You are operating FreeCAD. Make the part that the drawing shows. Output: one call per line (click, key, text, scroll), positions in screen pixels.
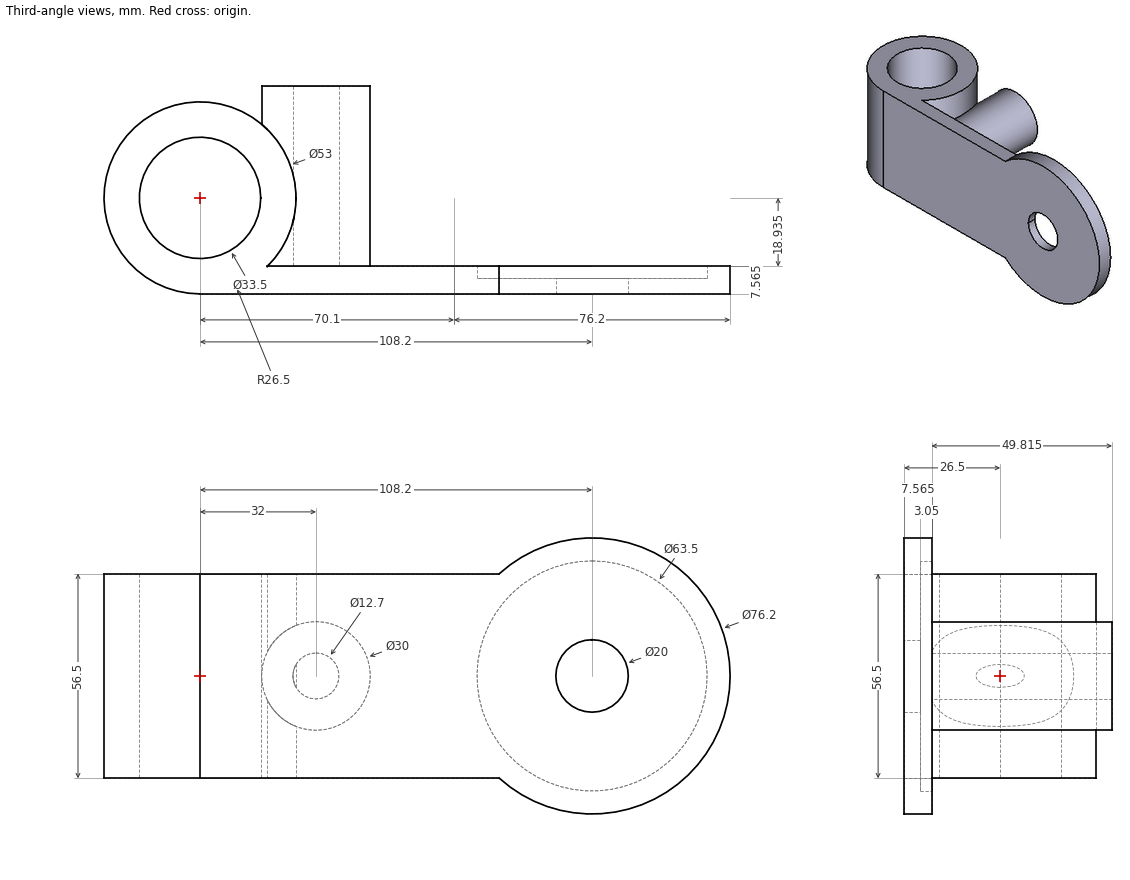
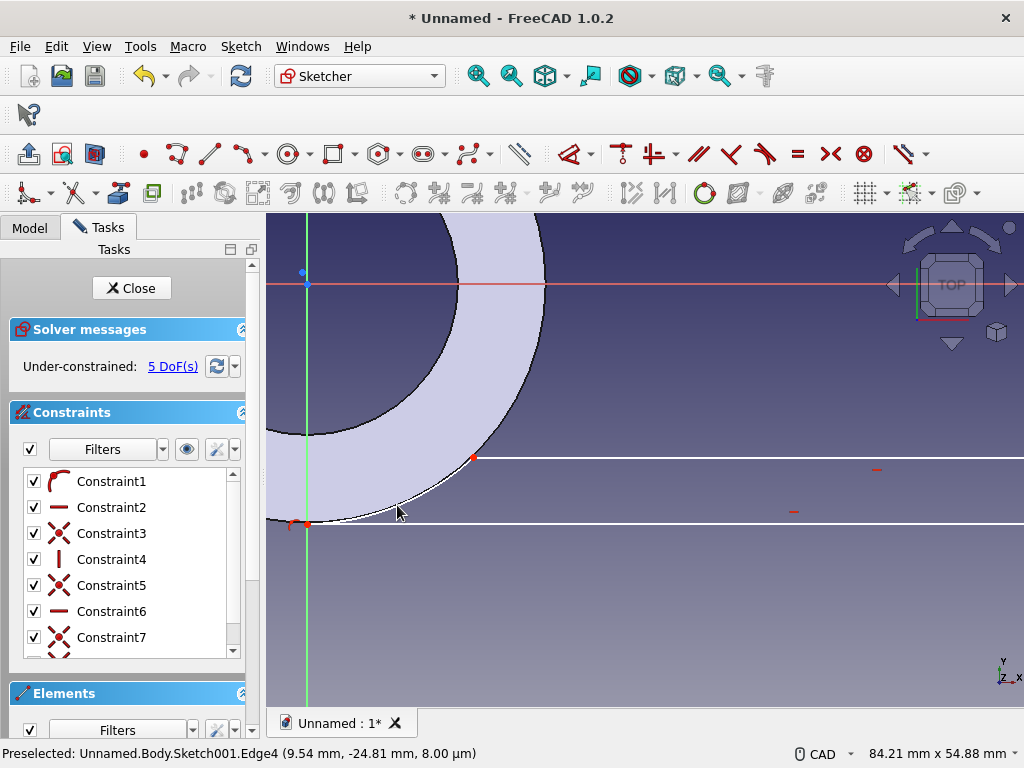
click(599, 524)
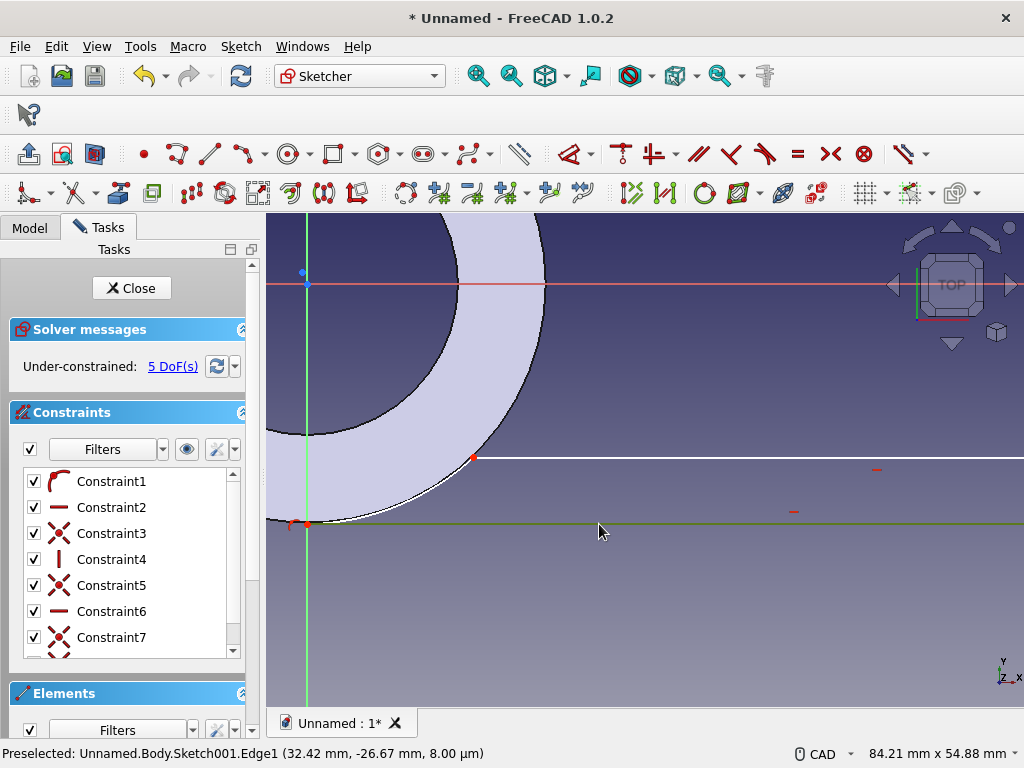
click(429, 490)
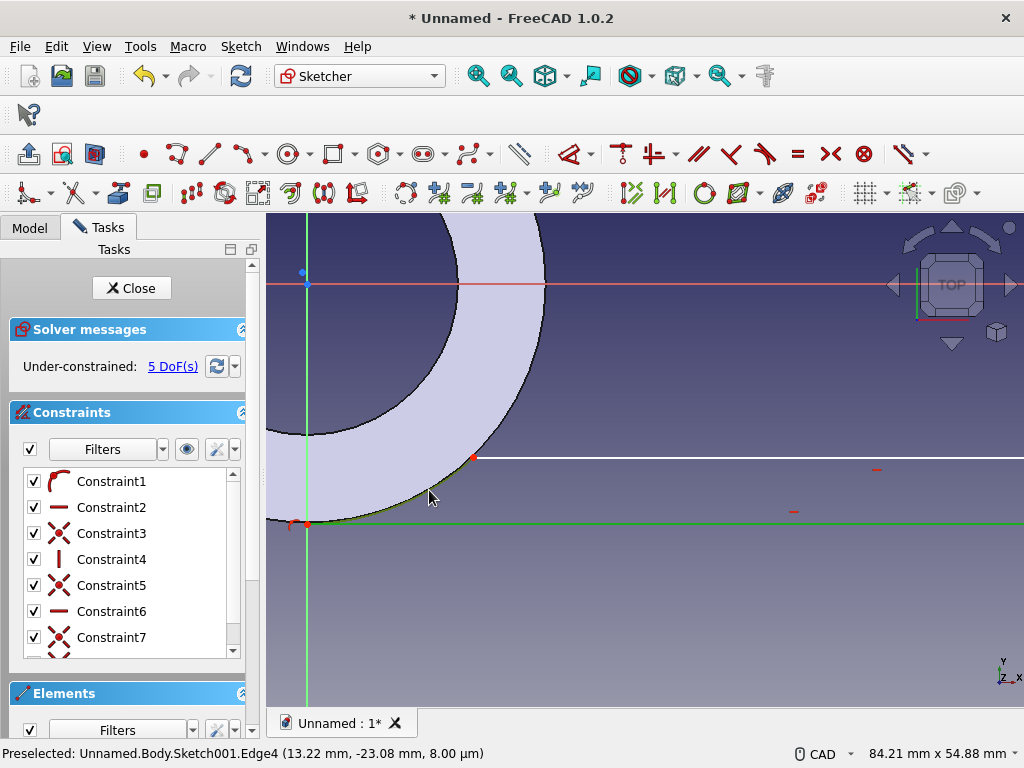
key(t)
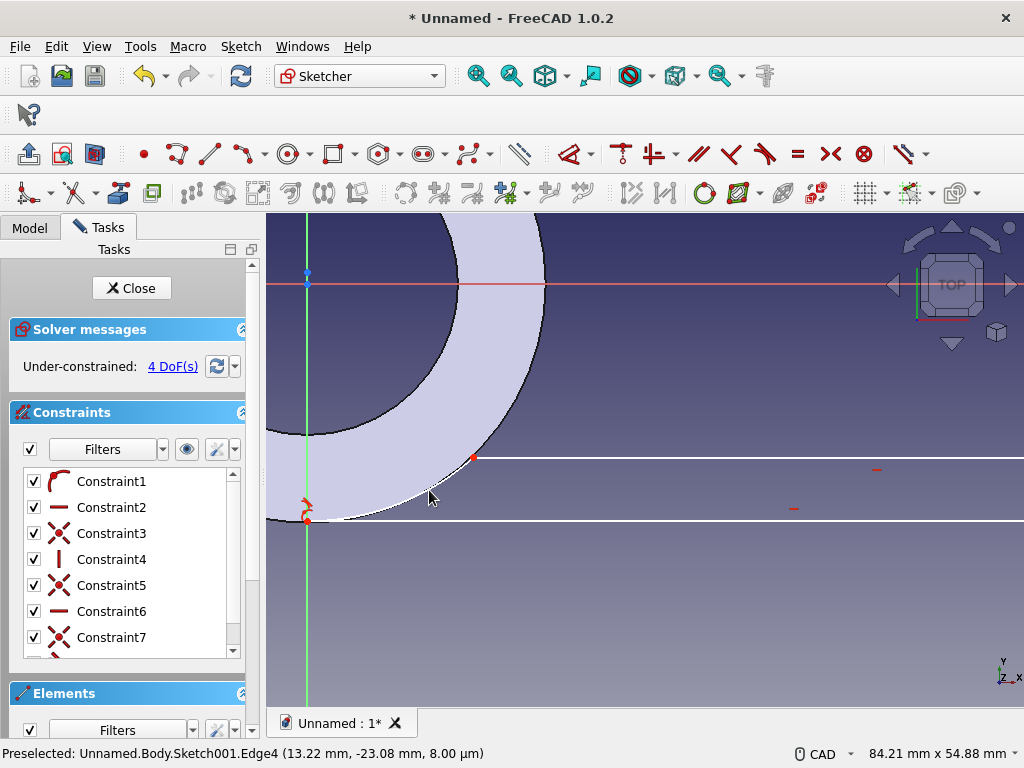
click(307, 273)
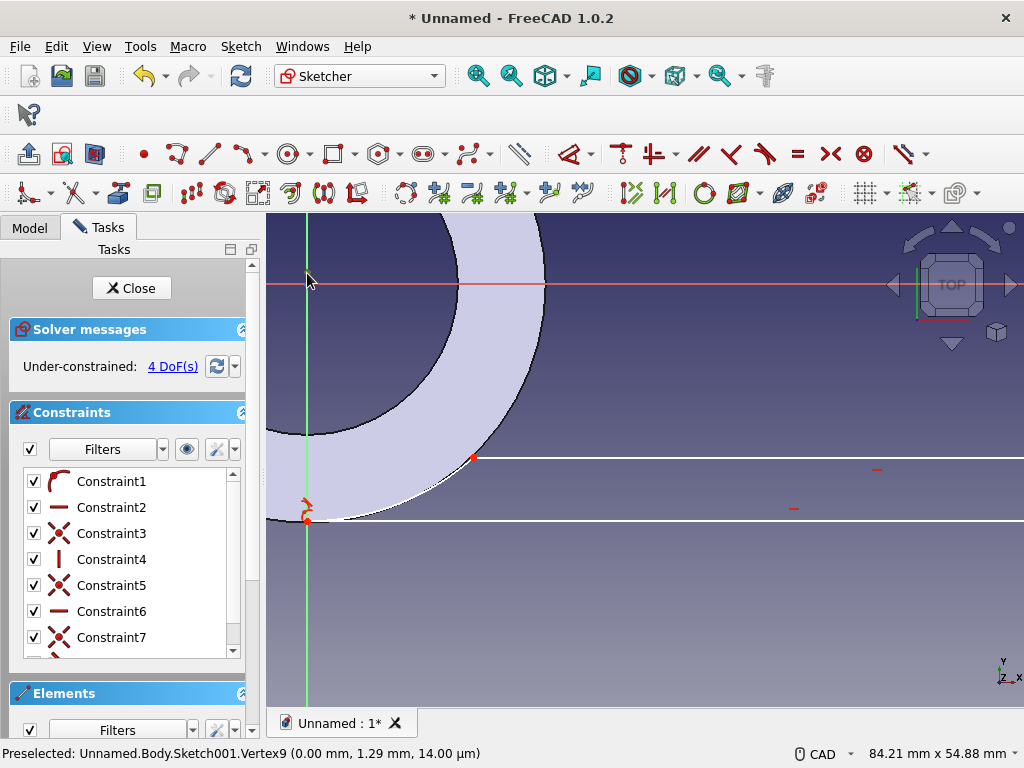
click(375, 284)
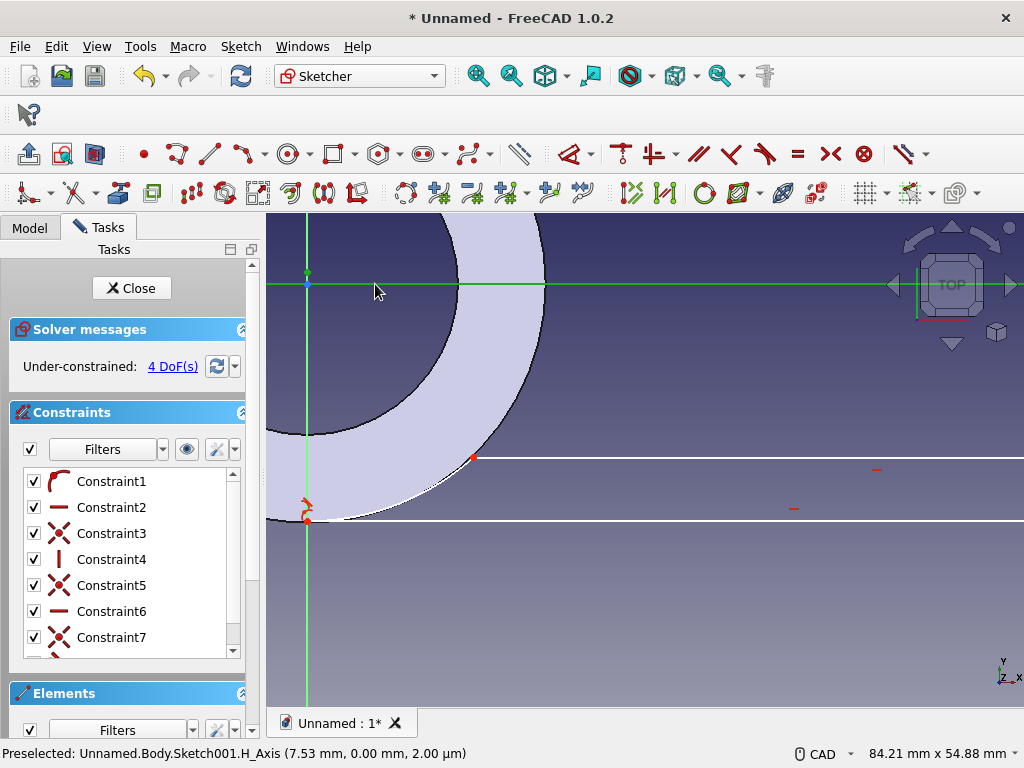
key(c)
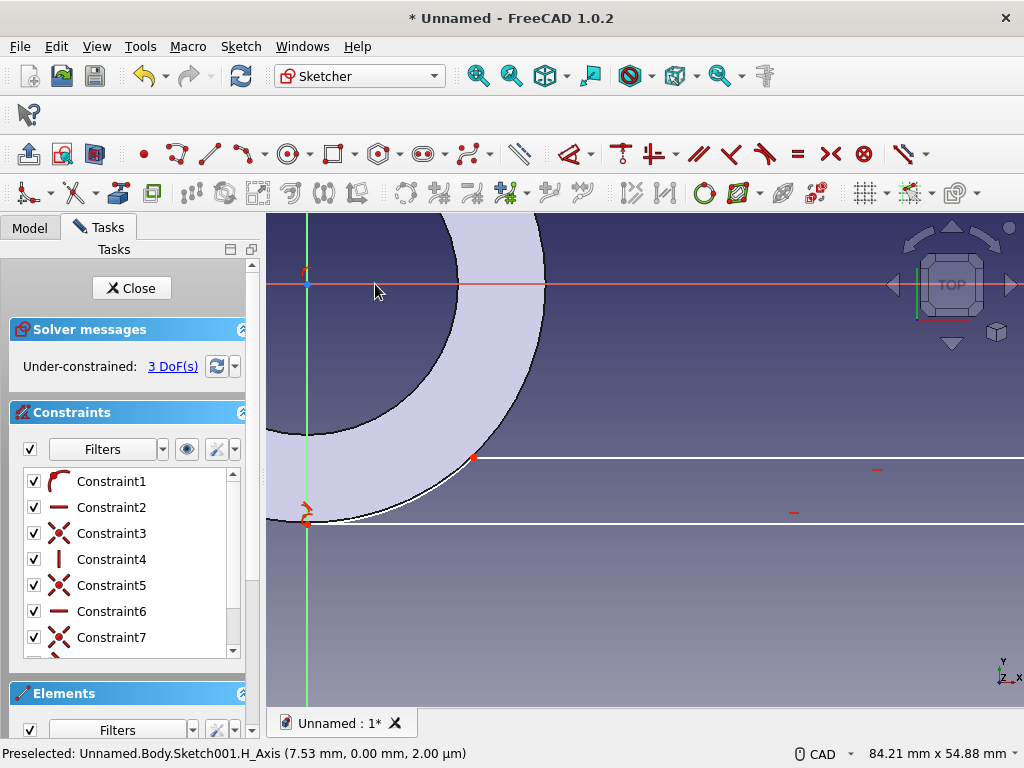
click(568, 154)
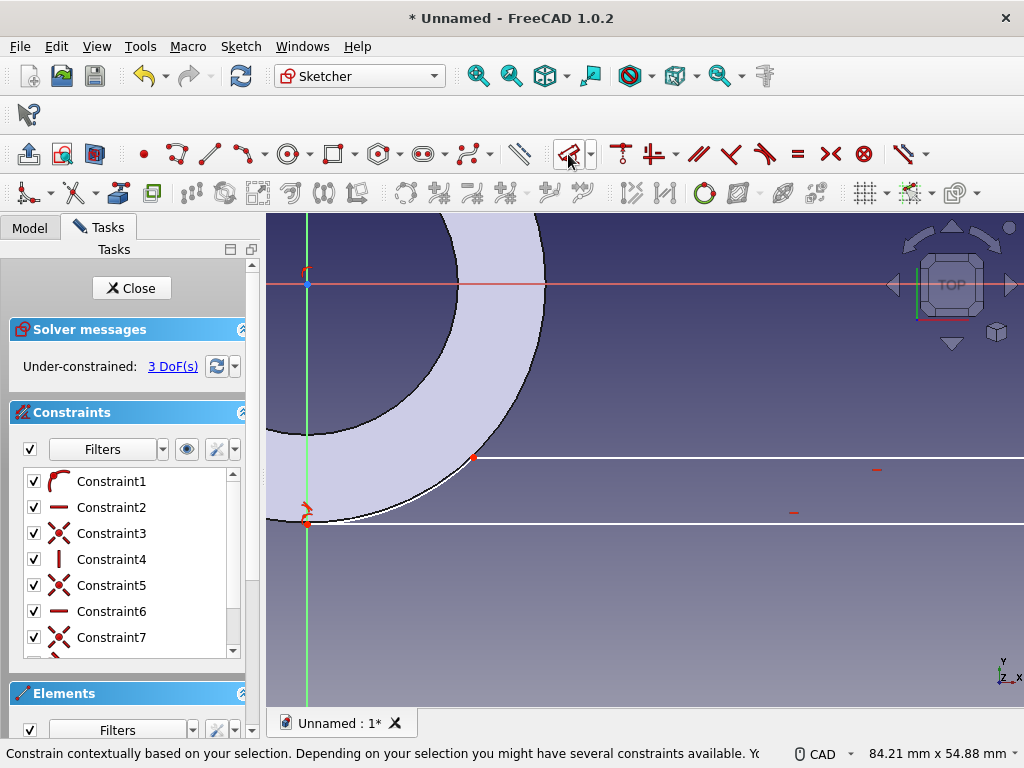
click(430, 491)
click(542, 423)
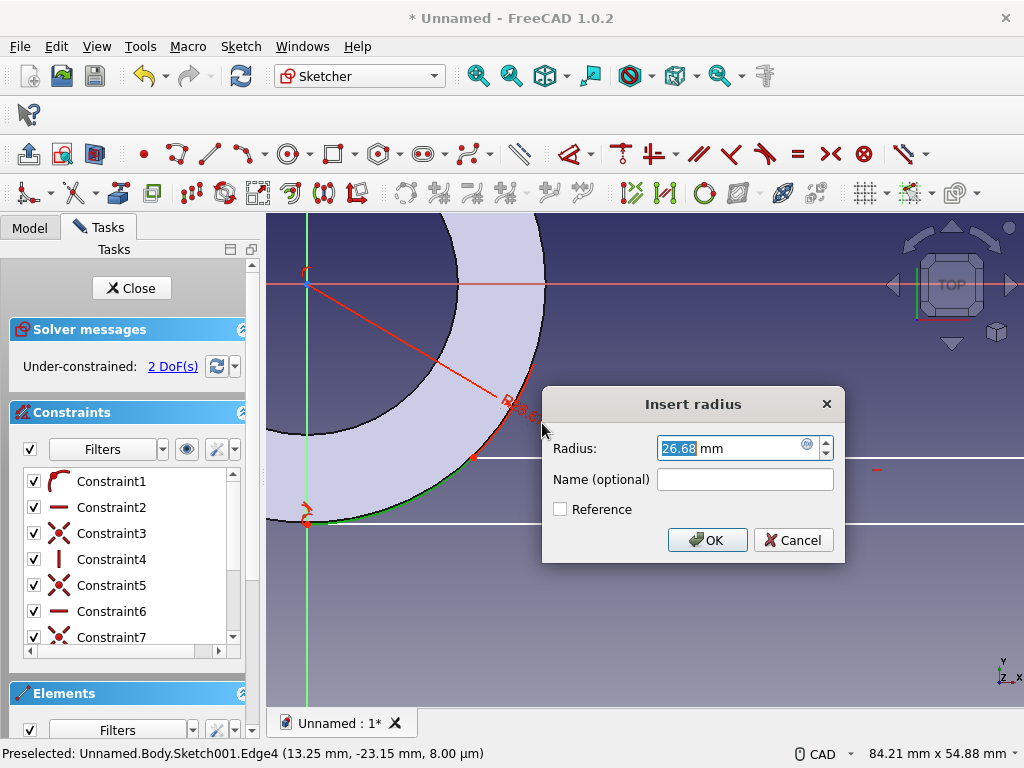
text(26.5)
key(Return)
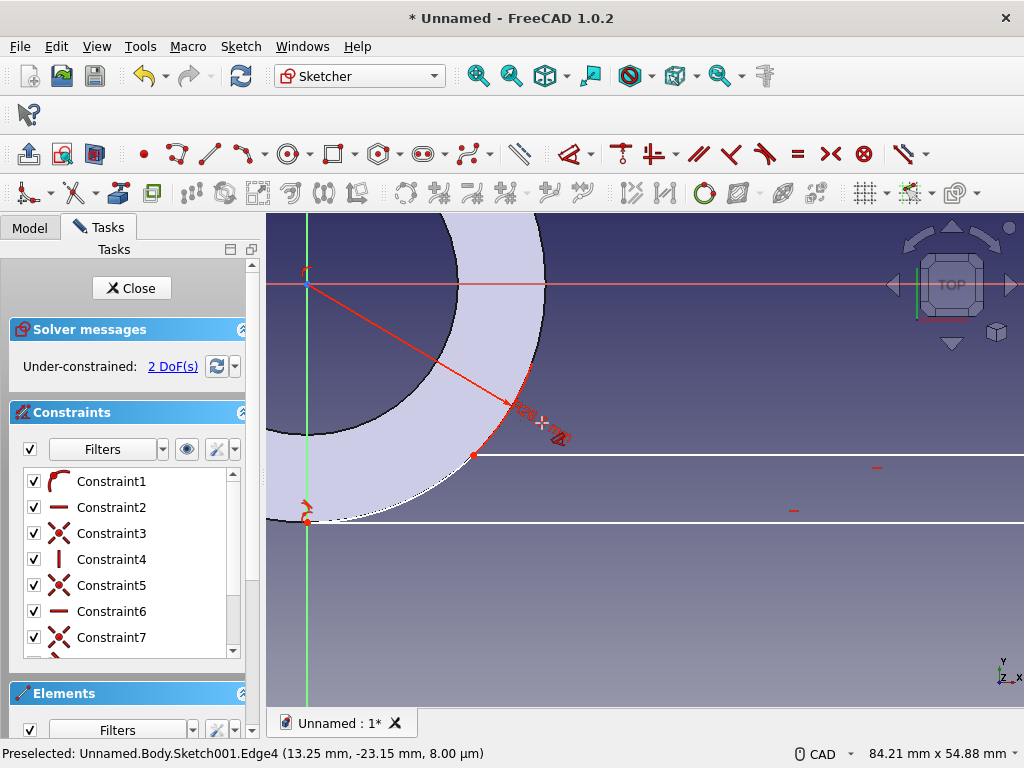
click(599, 523)
click(583, 557)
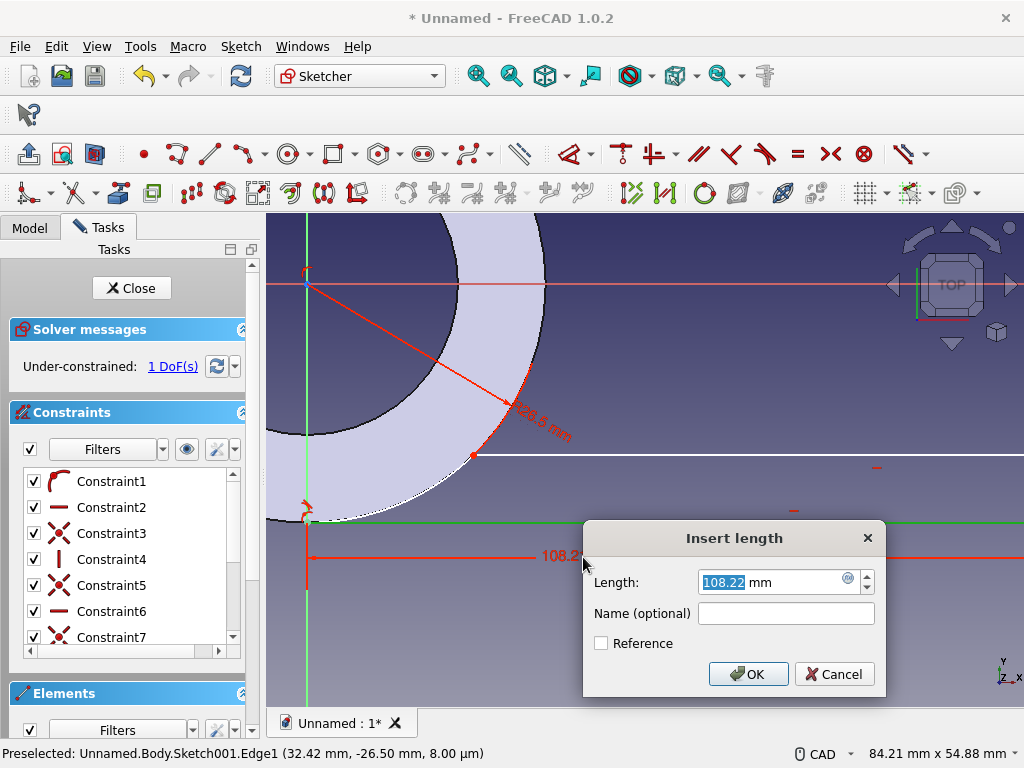
text(108.2)
key(Return)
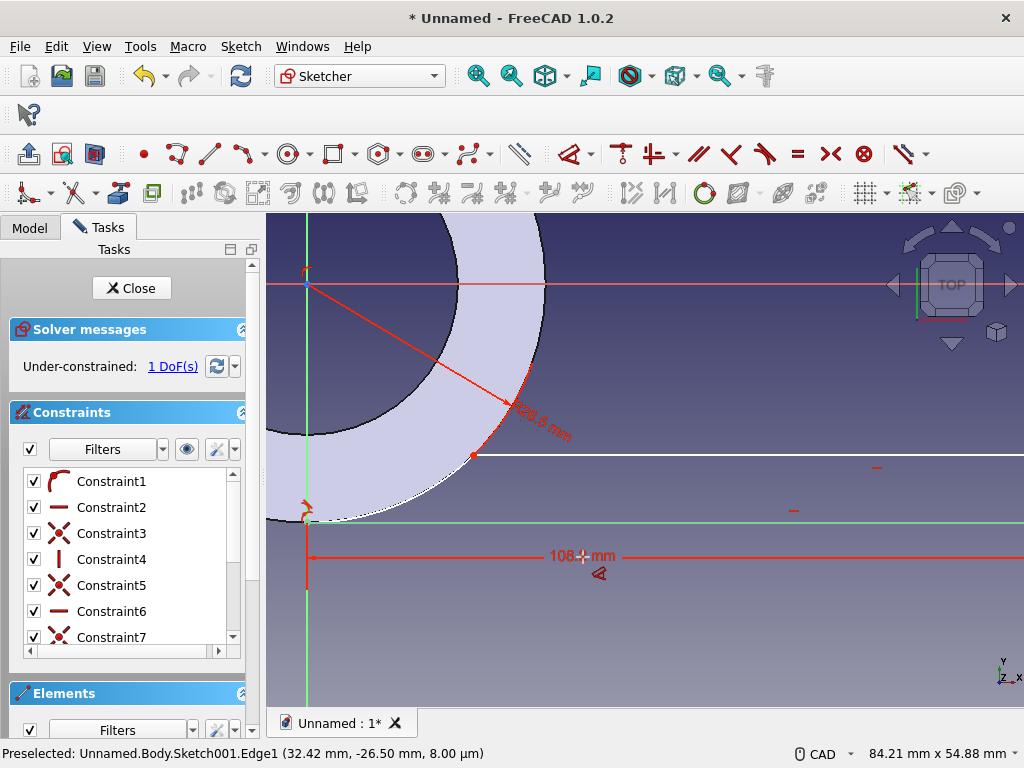
scroll(399, 506, down, 4)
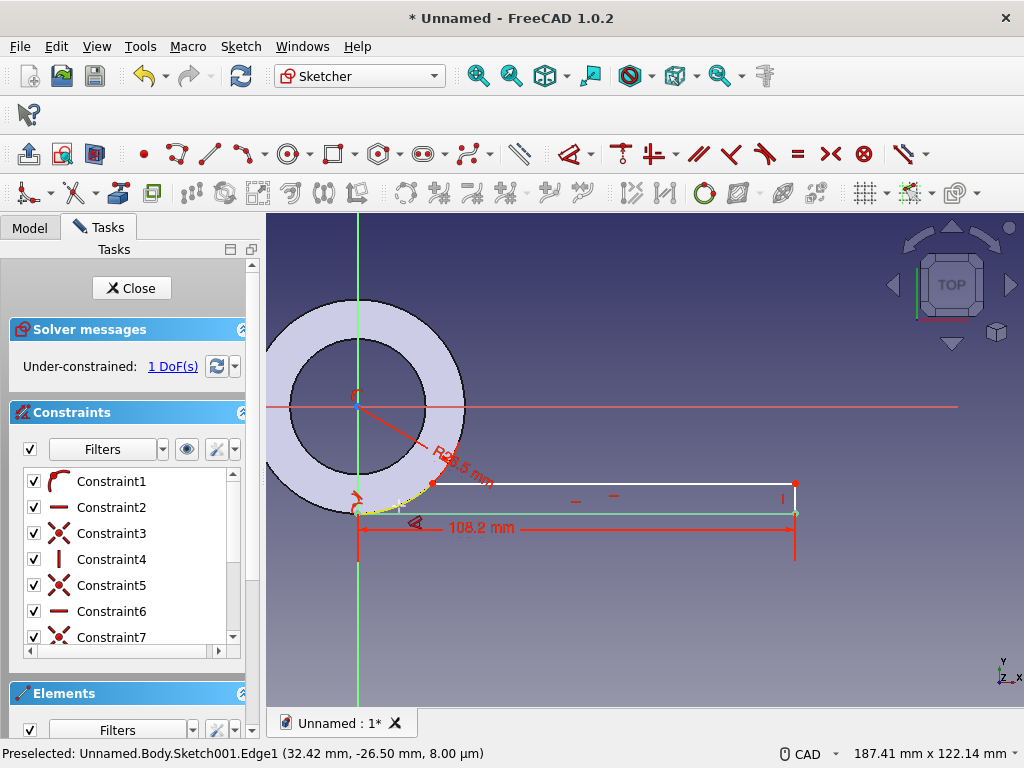
scroll(795, 505, up, 3)